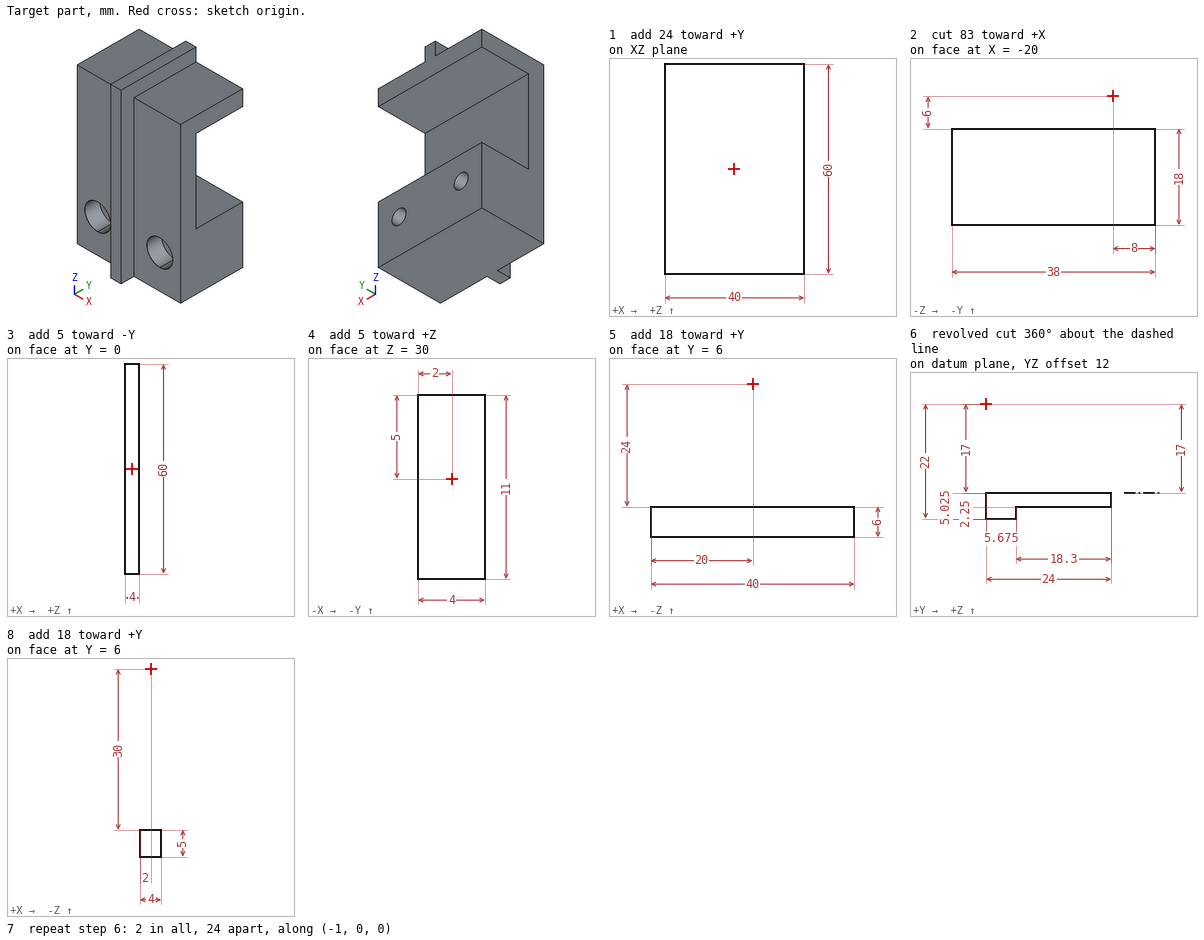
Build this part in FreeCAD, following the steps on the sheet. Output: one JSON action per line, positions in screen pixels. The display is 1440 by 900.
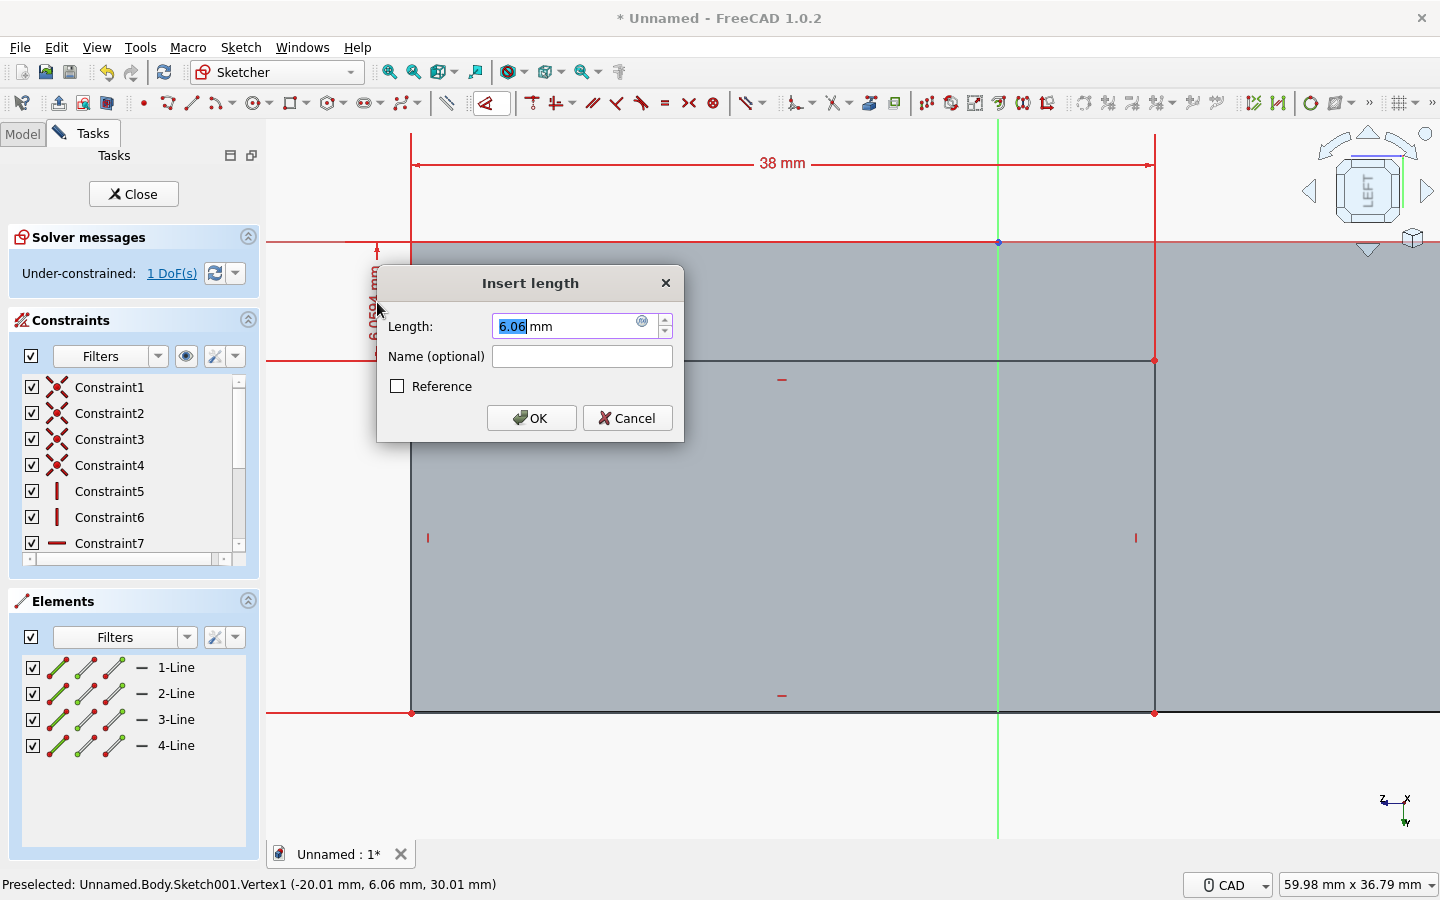
{"action": "type", "text": "6"}
{"action": "key", "text": "Return"}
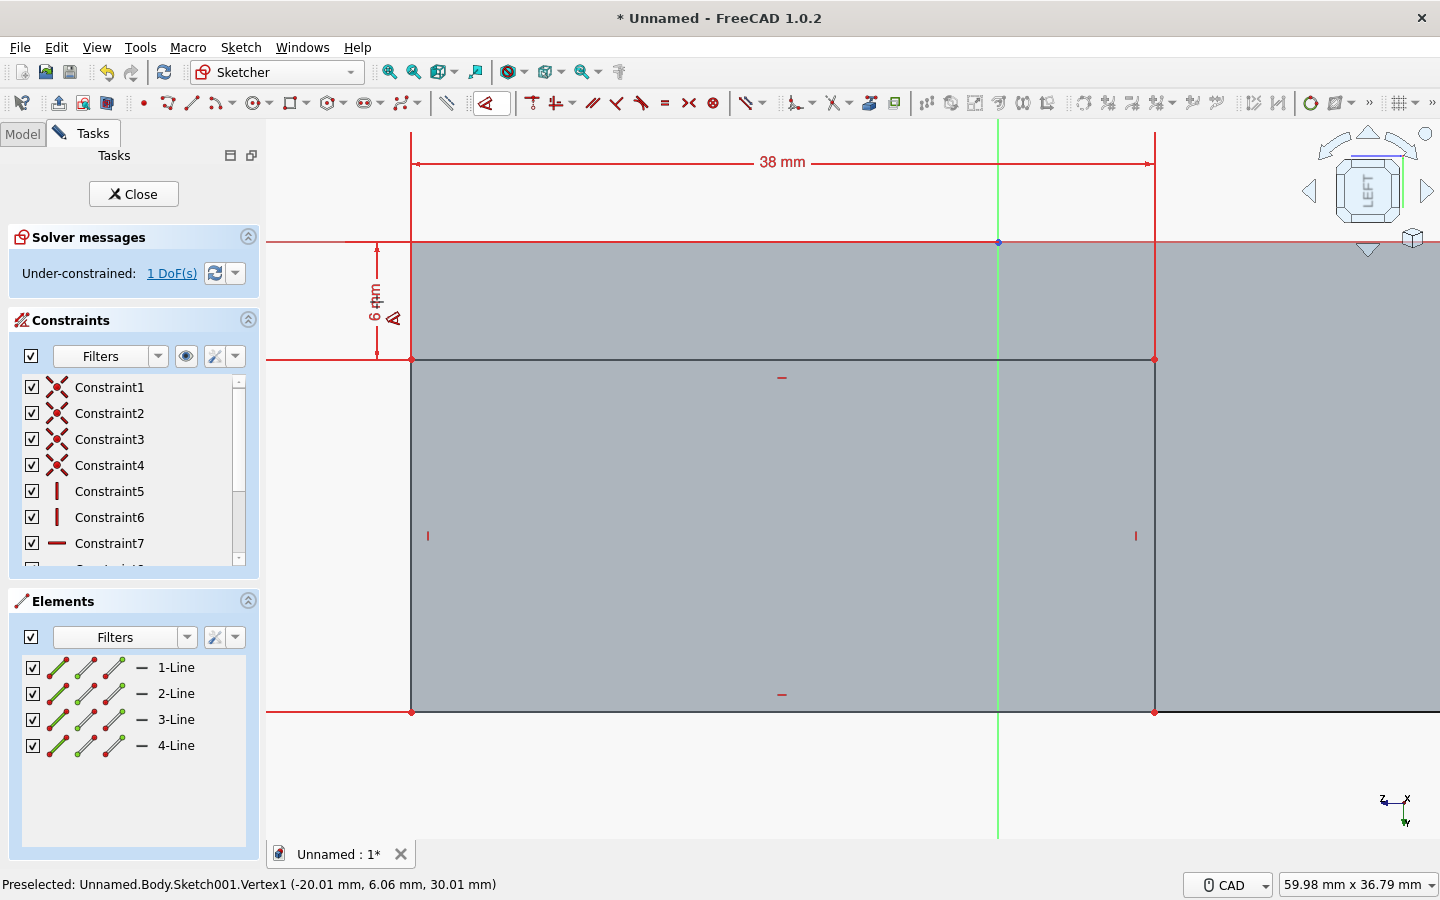
{"action": "left_click", "coordinate": [1155, 712]}
{"action": "left_click", "coordinate": [1077, 746]}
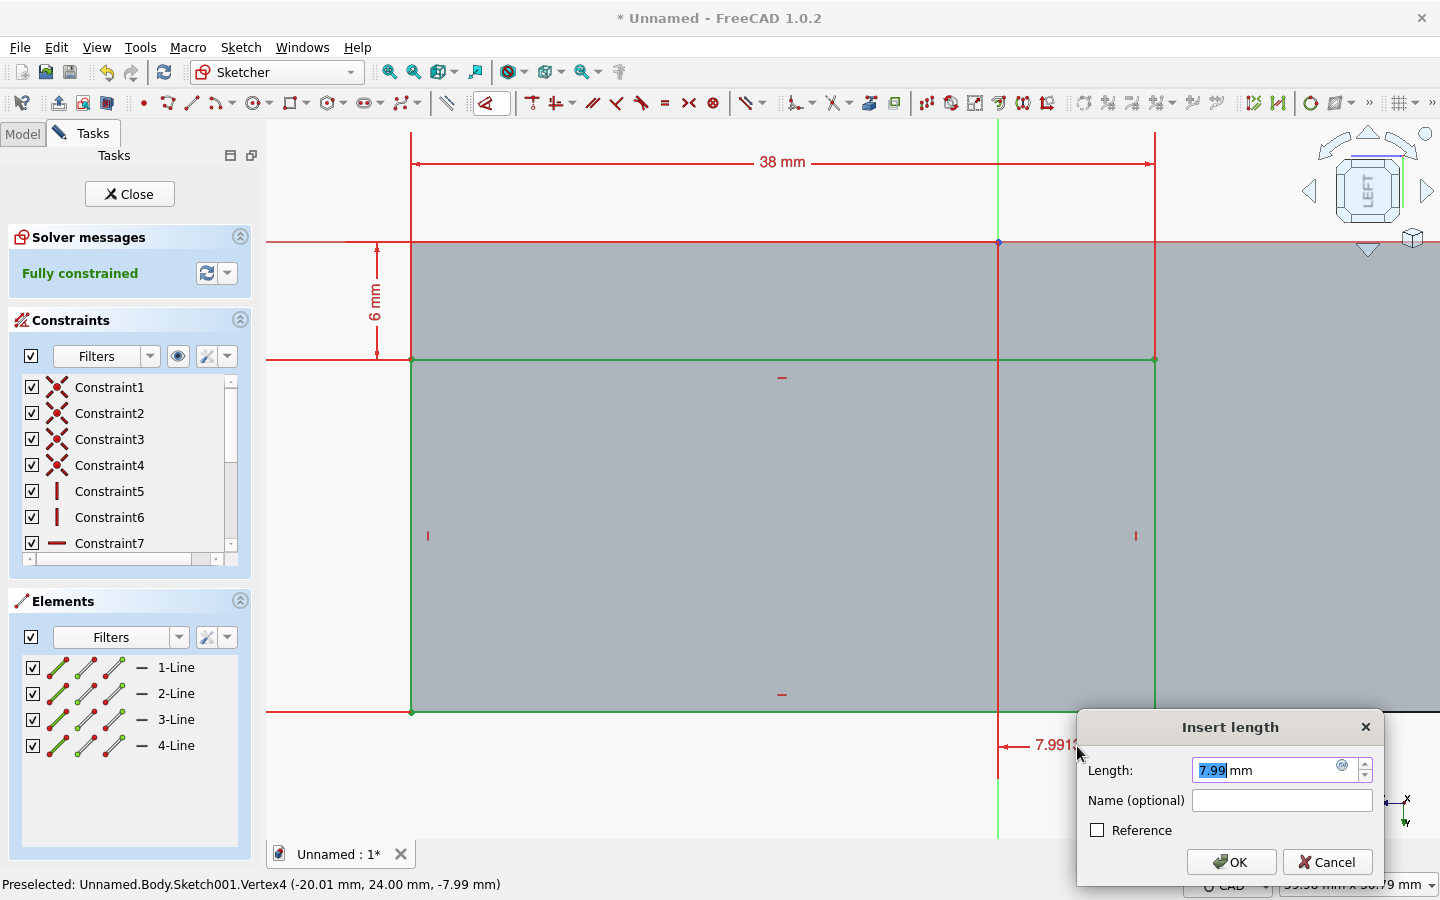
{"action": "type", "text": "8"}
{"action": "key", "text": "Return"}
{"action": "key", "text": "Escape"}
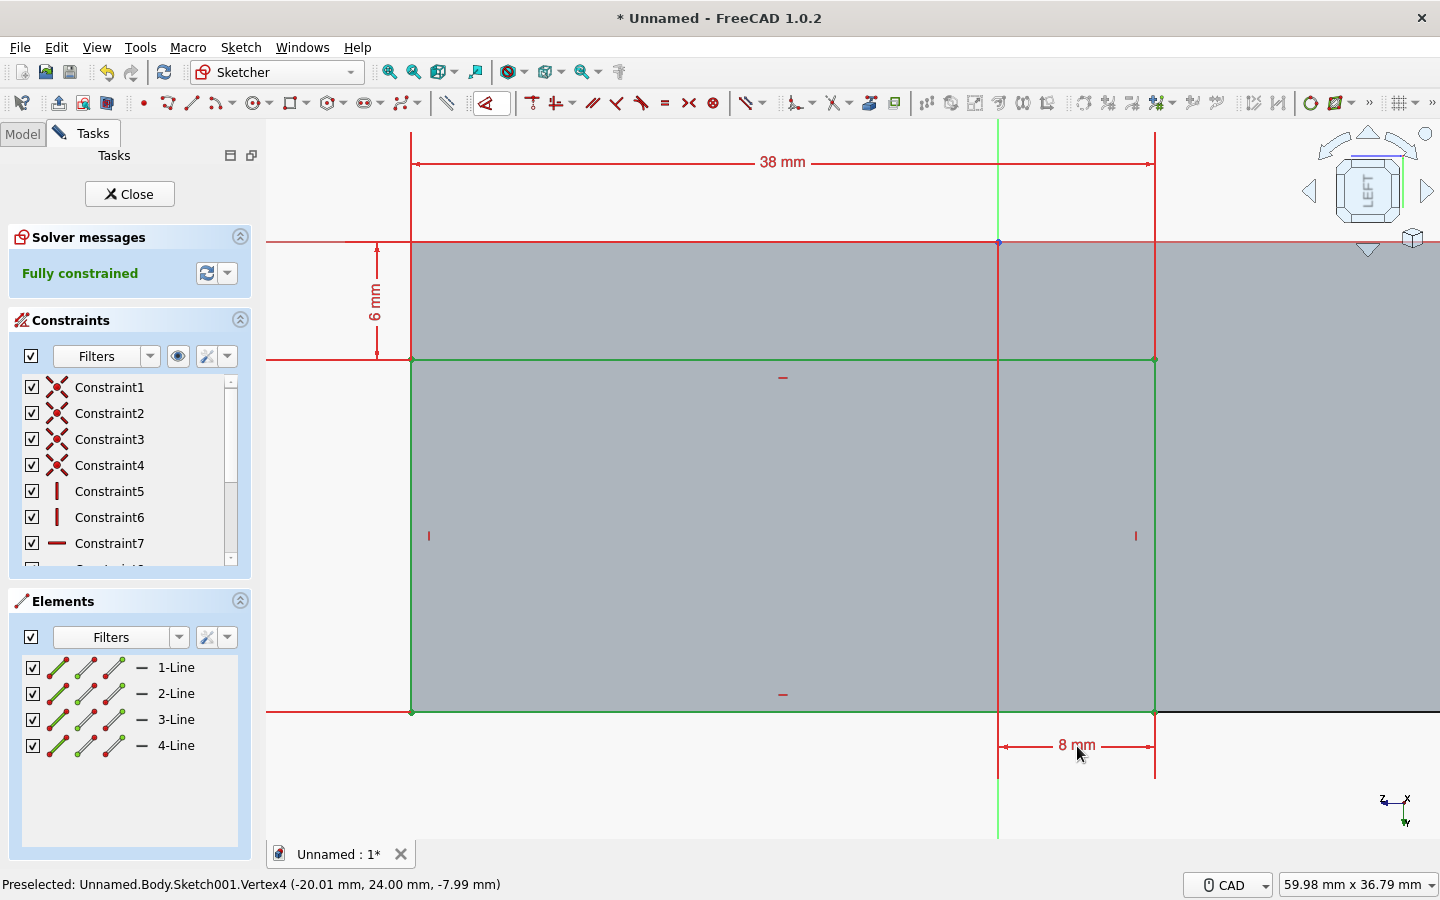
{"action": "left_click", "coordinate": [130, 194]}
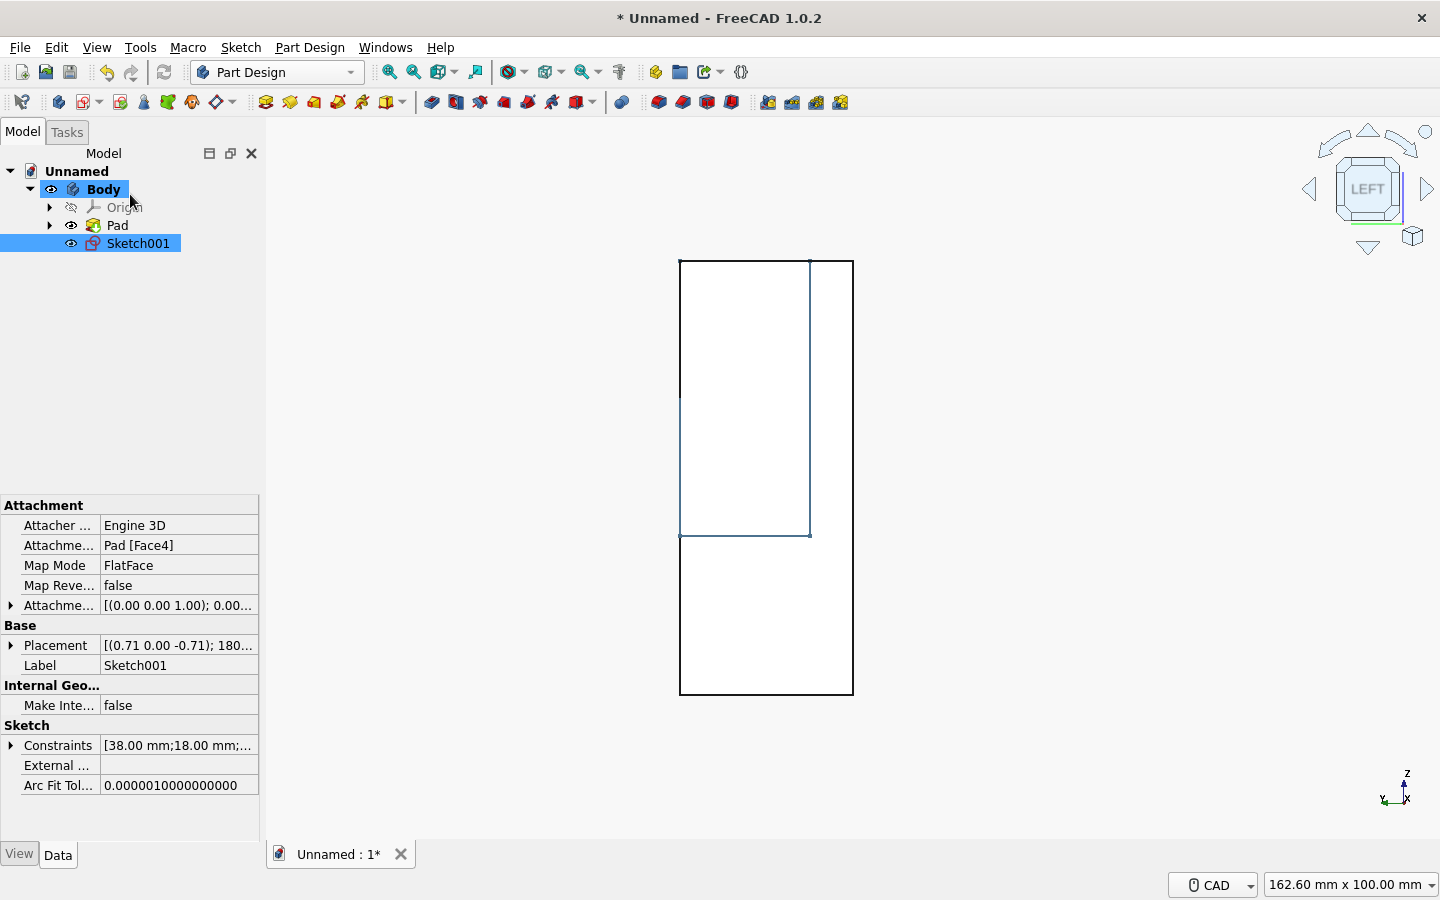
{"action": "left_click", "coordinate": [432, 102]}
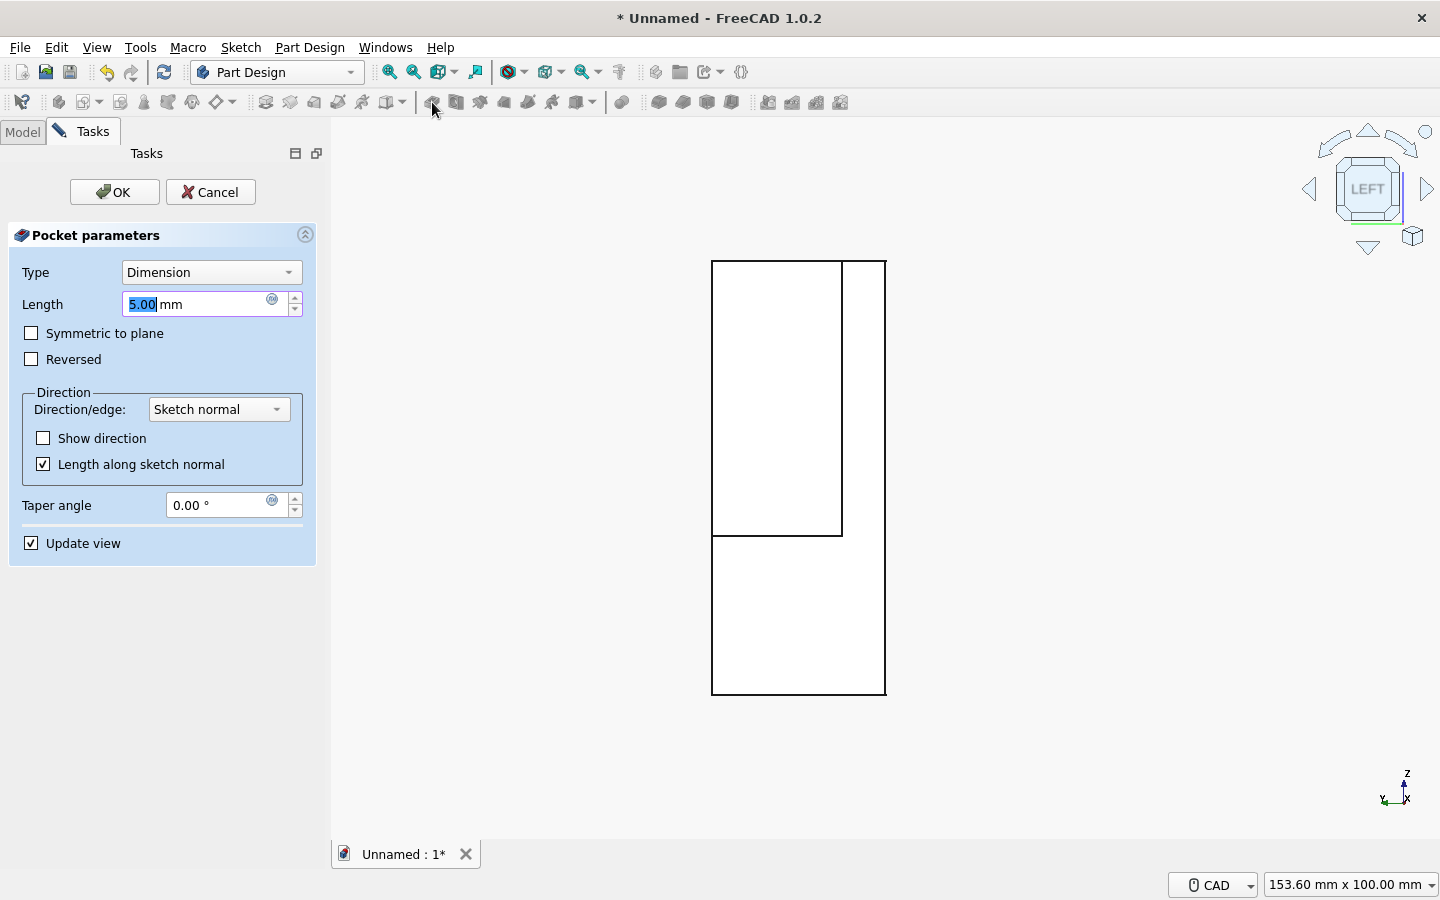
{"action": "type", "text": "83"}
{"action": "key", "text": "Tab"}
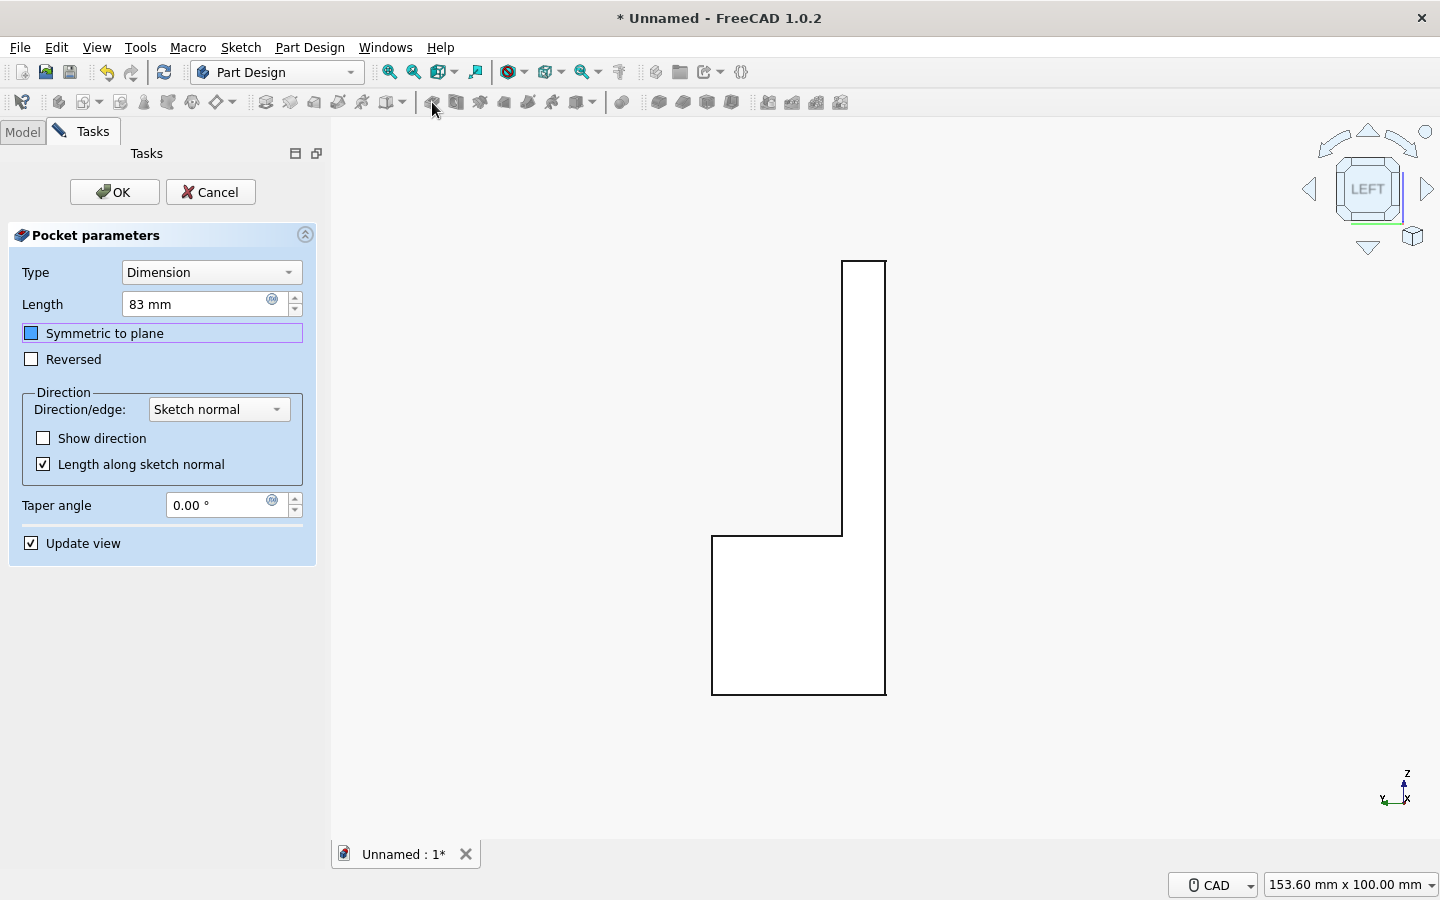
{"action": "left_click", "coordinate": [115, 192]}